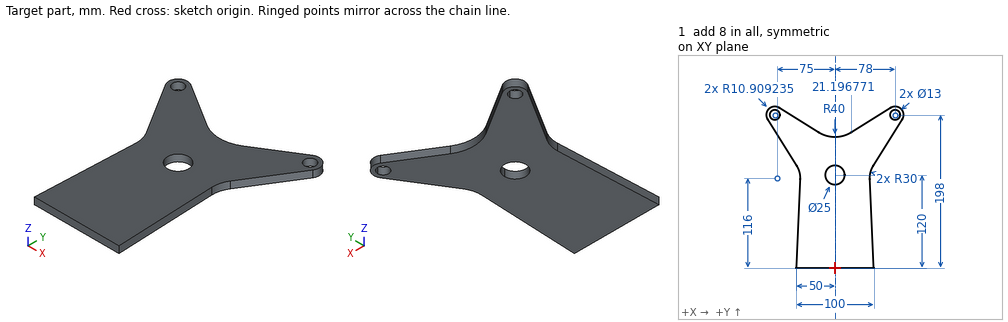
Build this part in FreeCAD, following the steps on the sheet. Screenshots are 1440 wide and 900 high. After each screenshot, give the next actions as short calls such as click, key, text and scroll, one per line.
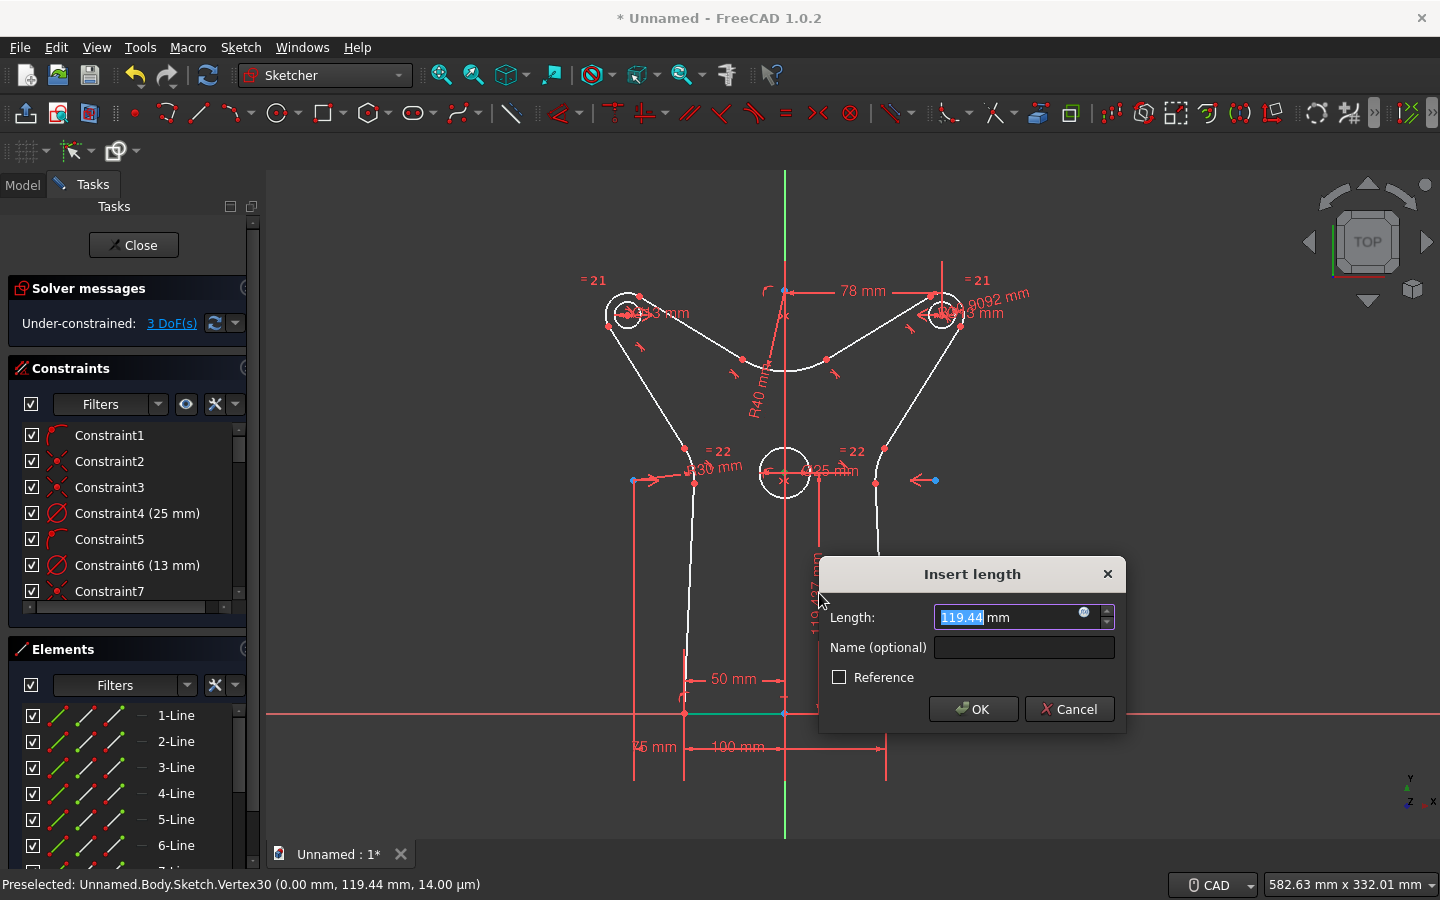
text(120)
key(Return)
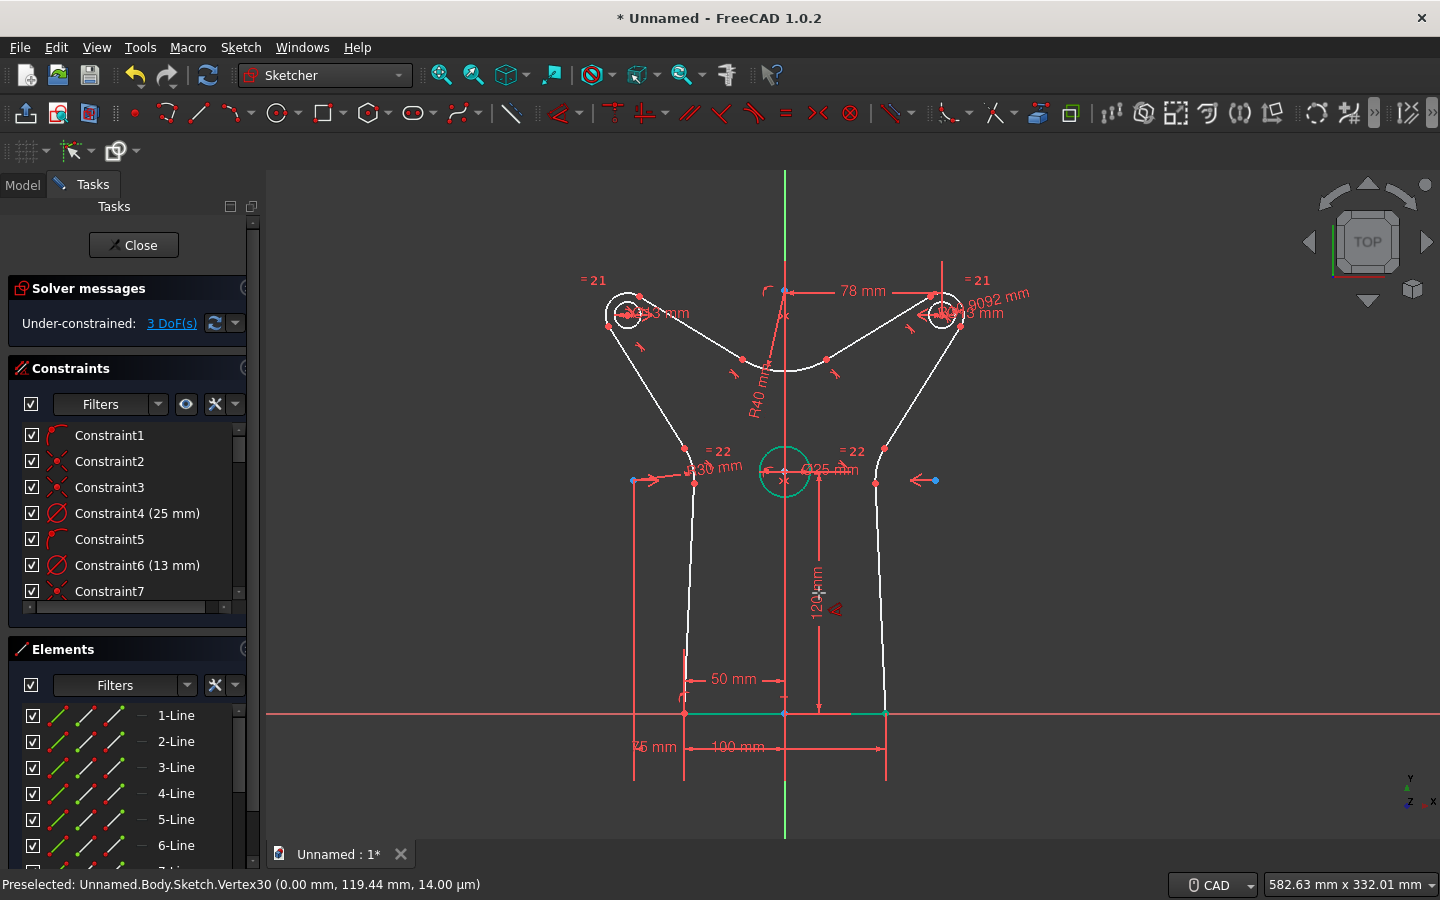
click(942, 315)
click(976, 514)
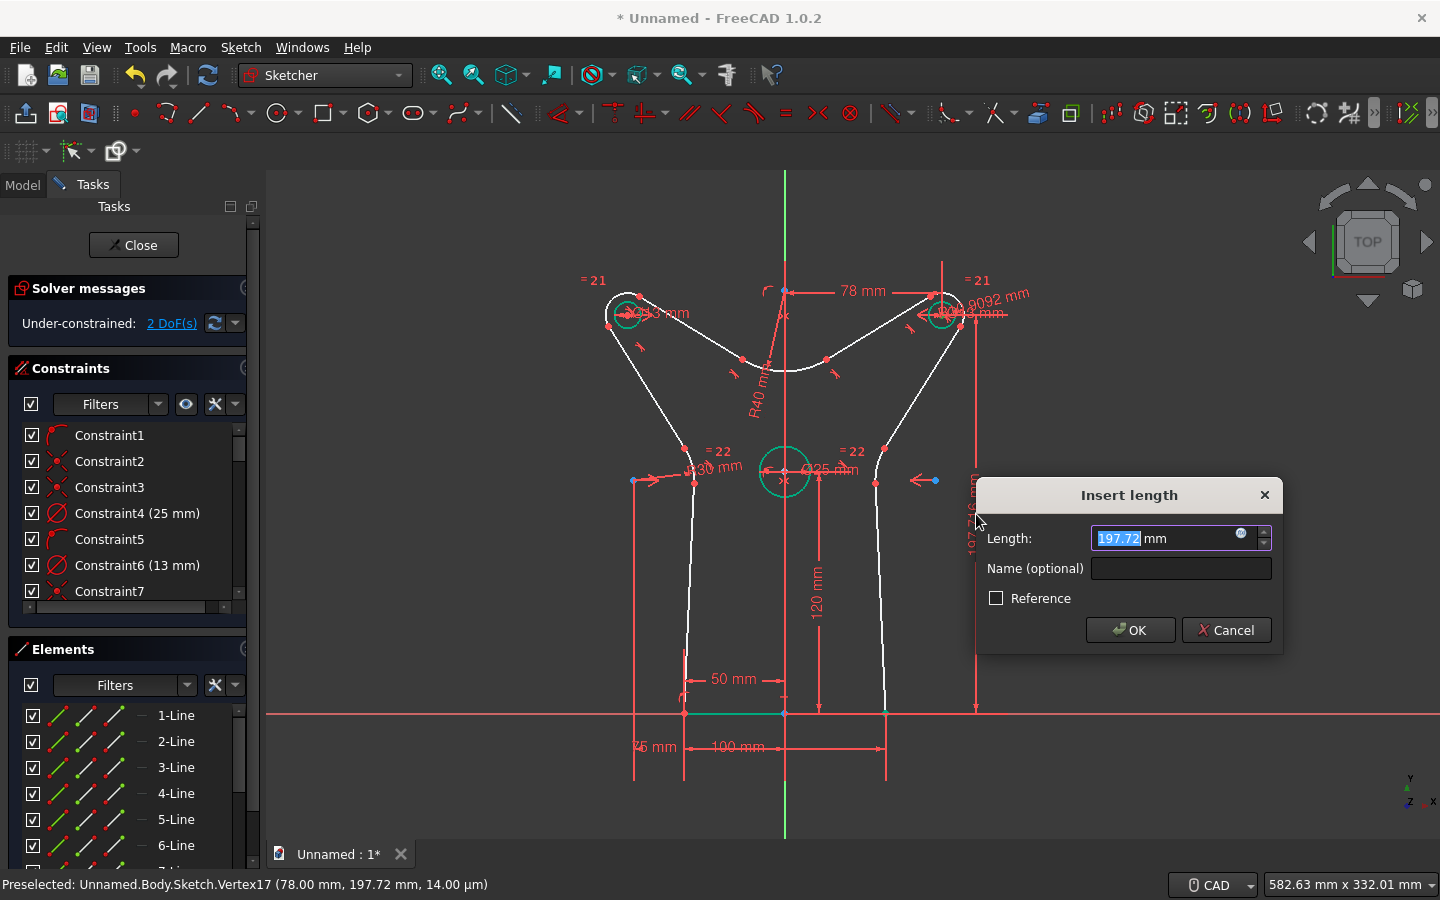
text(198)
key(Return)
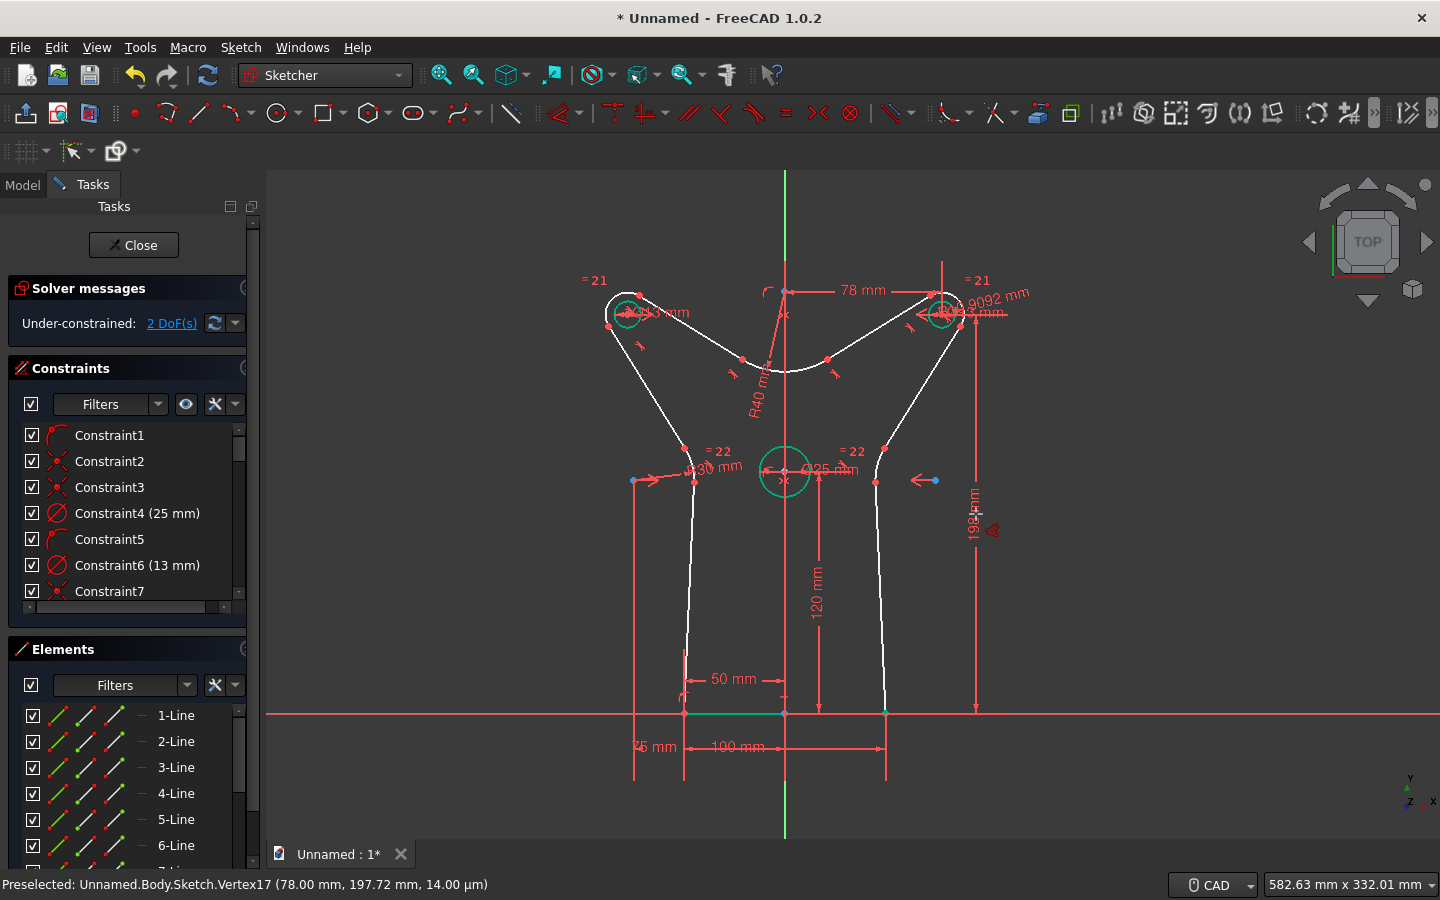
click(634, 480)
click(600, 597)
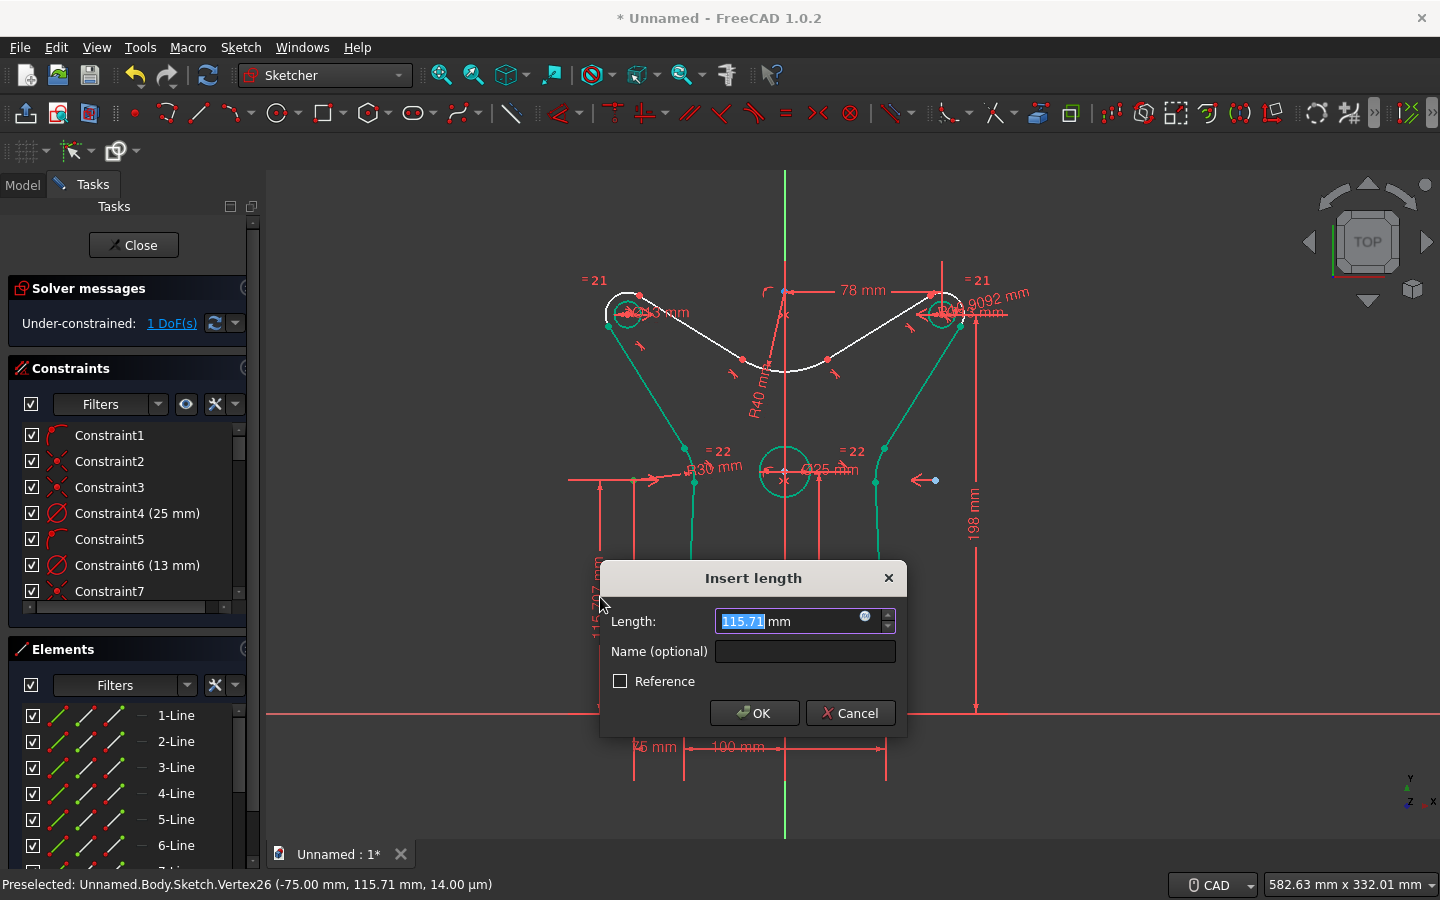
text(116)
key(Return)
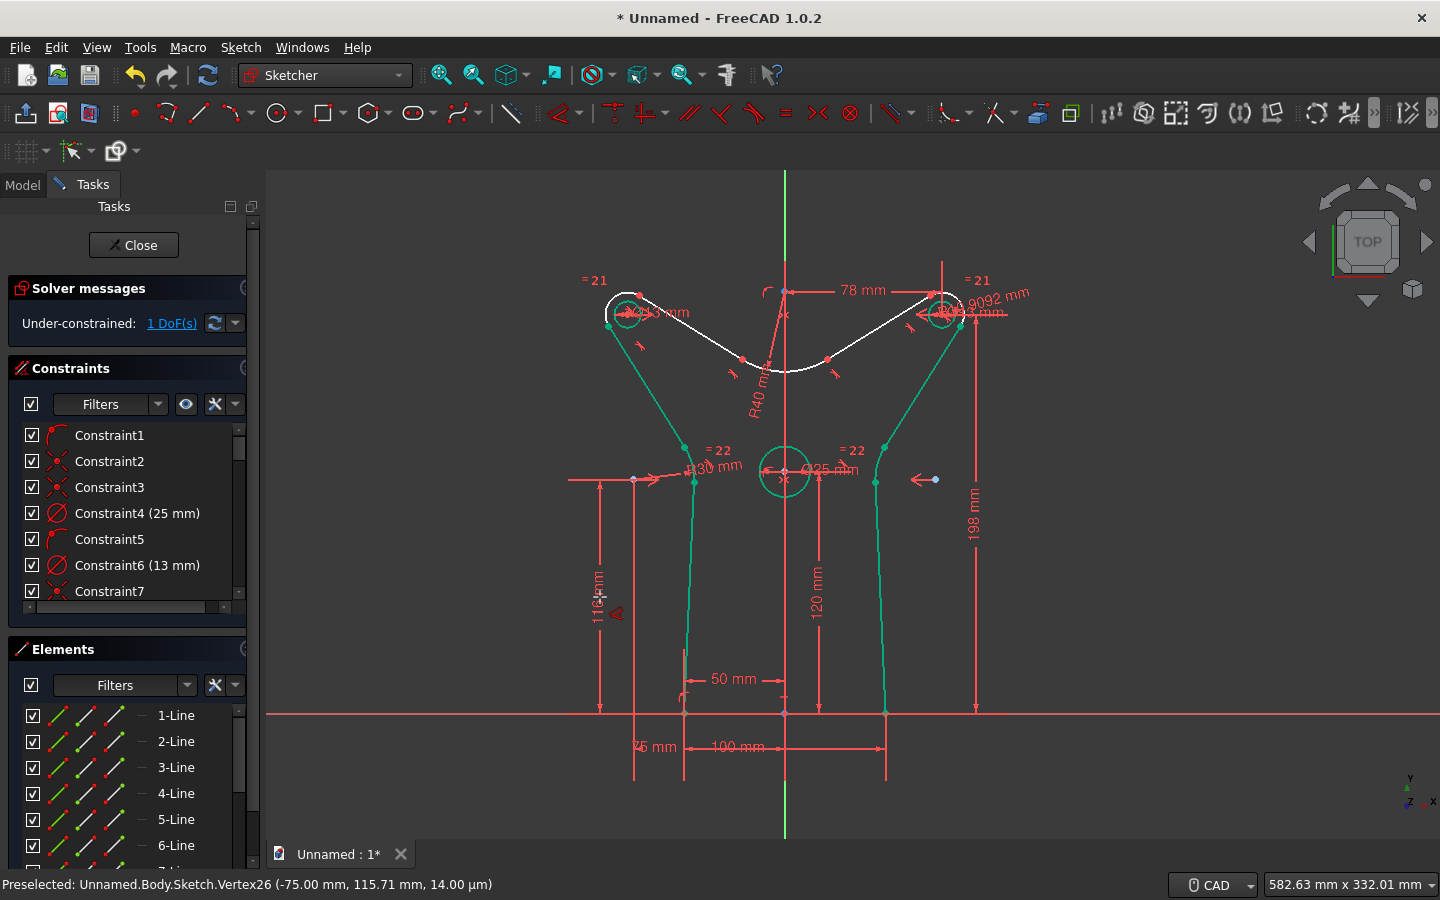
click(827, 360)
click(816, 748)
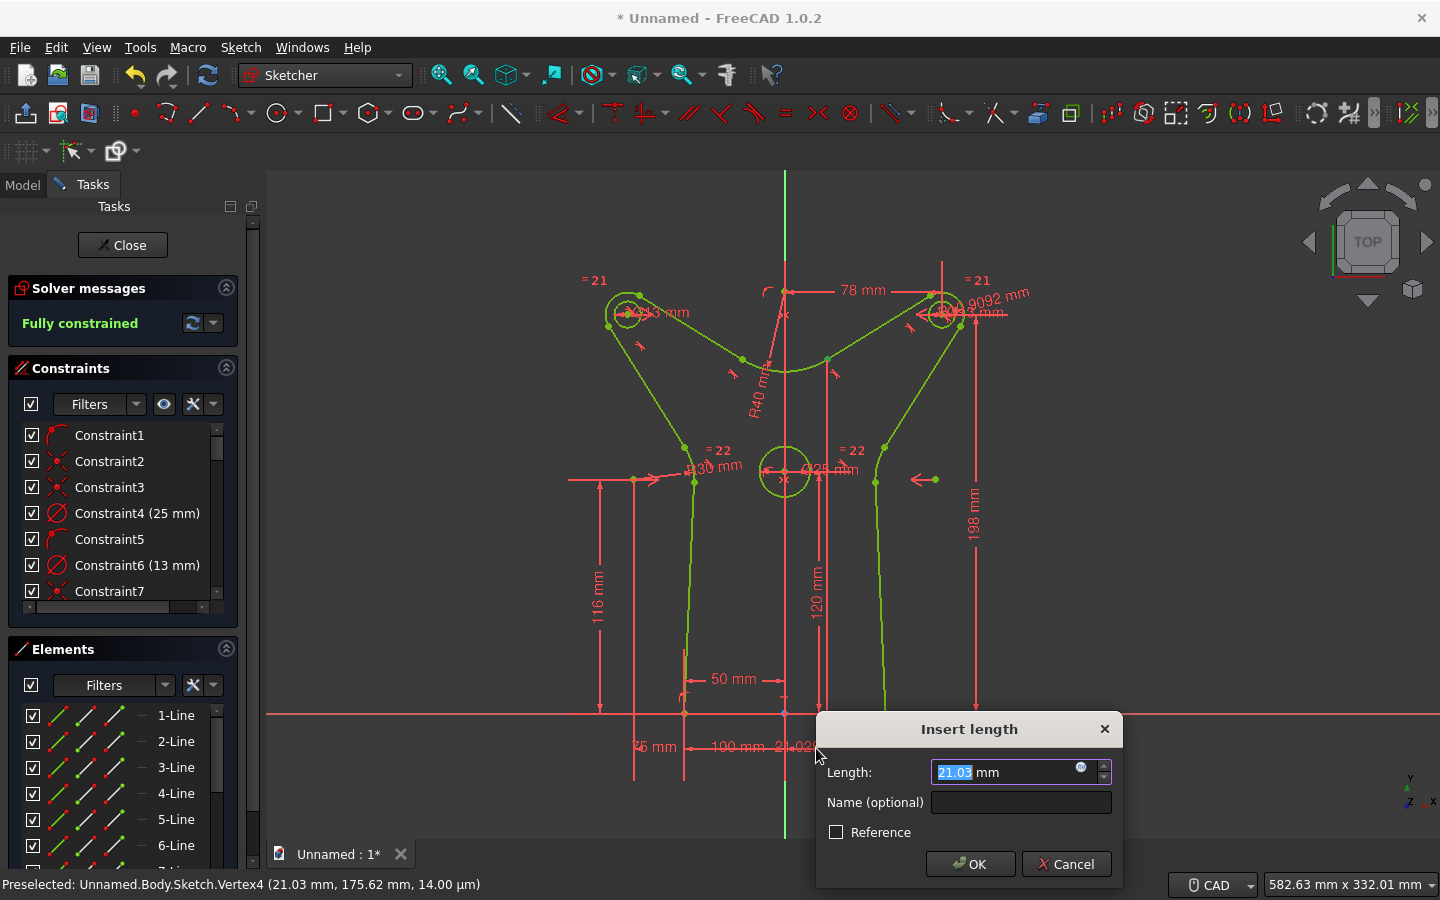
text(21.196771)
key(Return)
key(Escape)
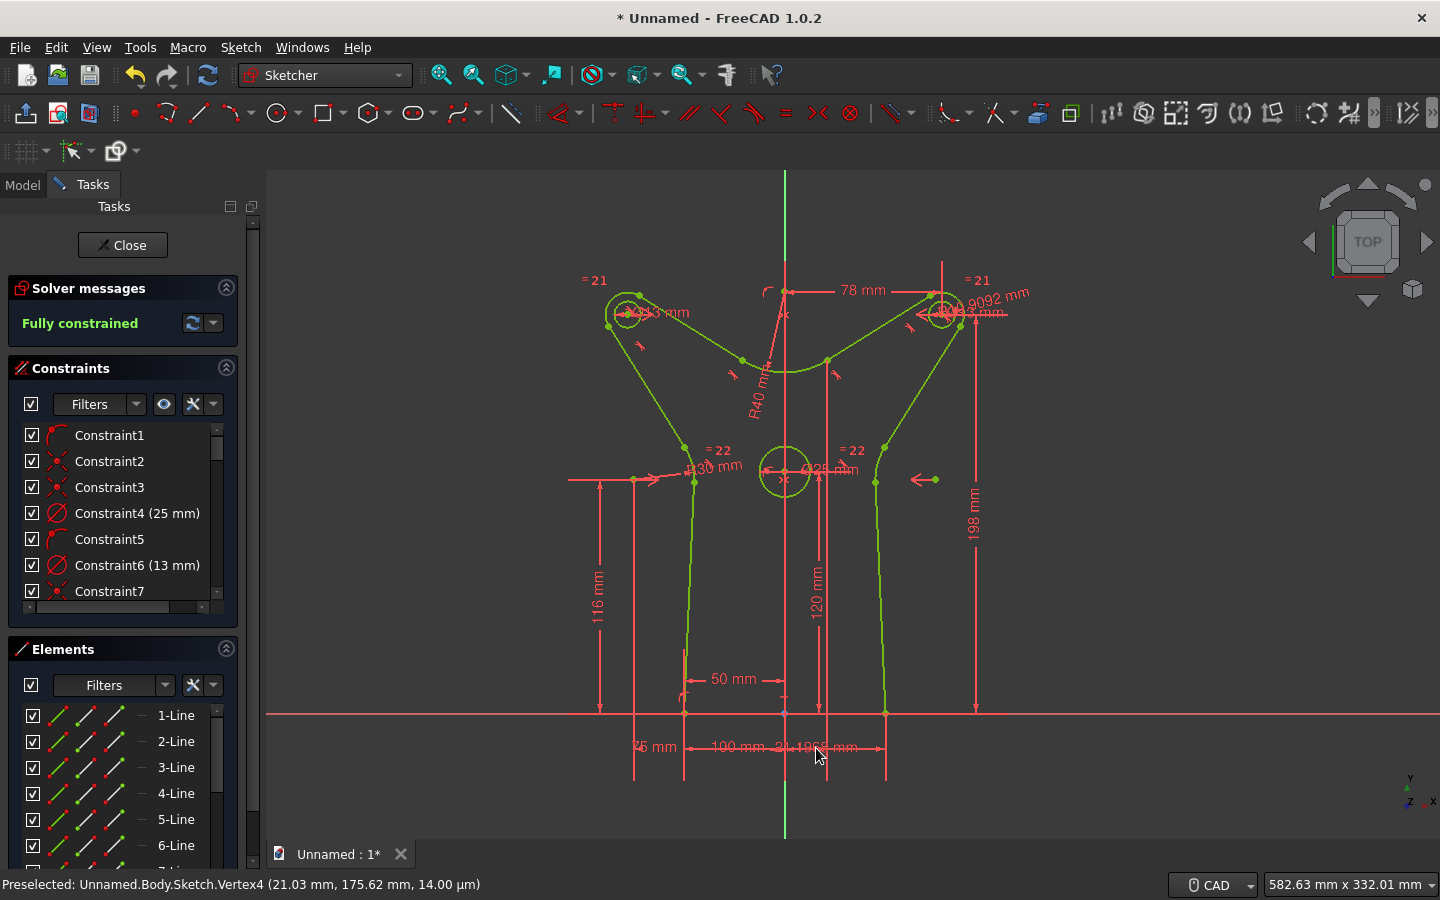
click(123, 245)